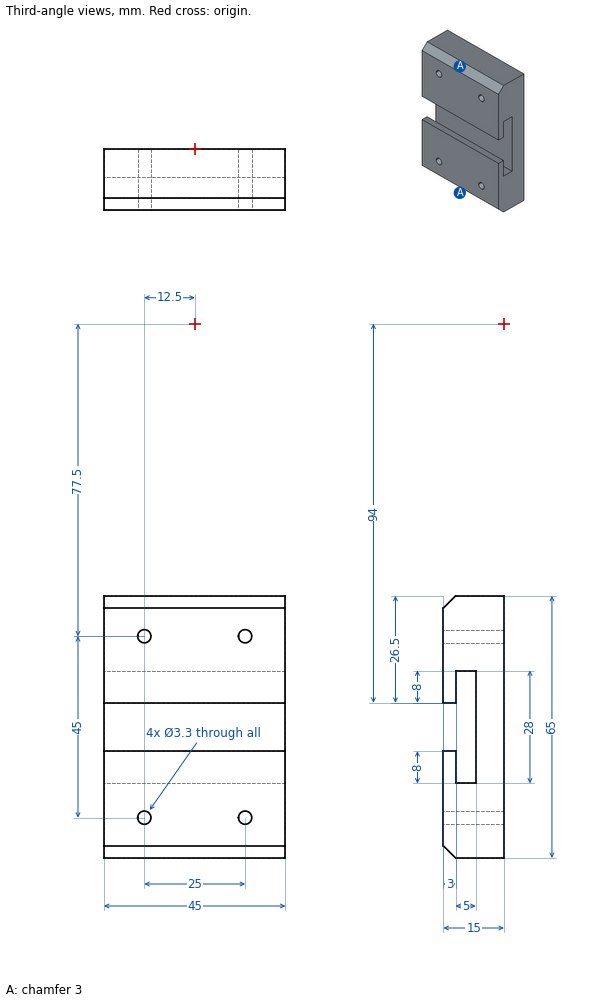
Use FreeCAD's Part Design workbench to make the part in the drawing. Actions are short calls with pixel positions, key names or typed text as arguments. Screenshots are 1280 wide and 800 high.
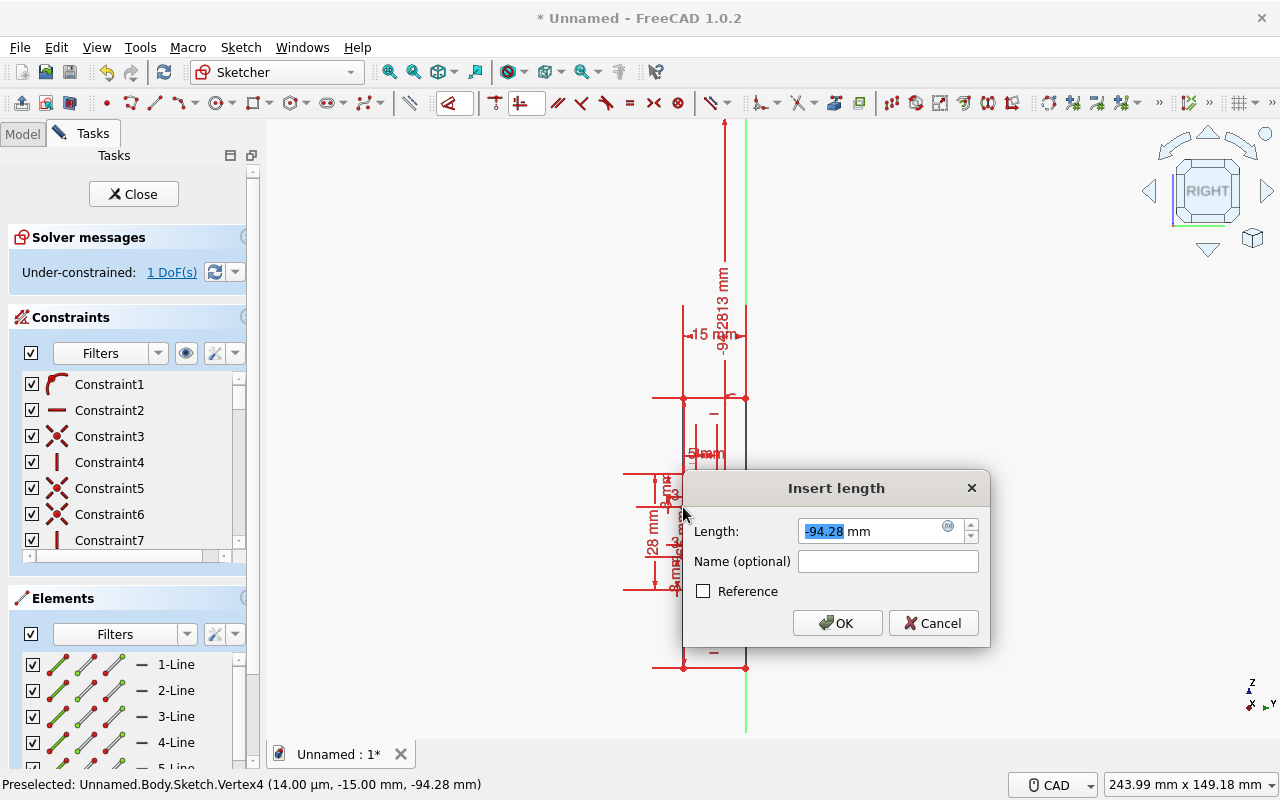
text(-94)
key(Return)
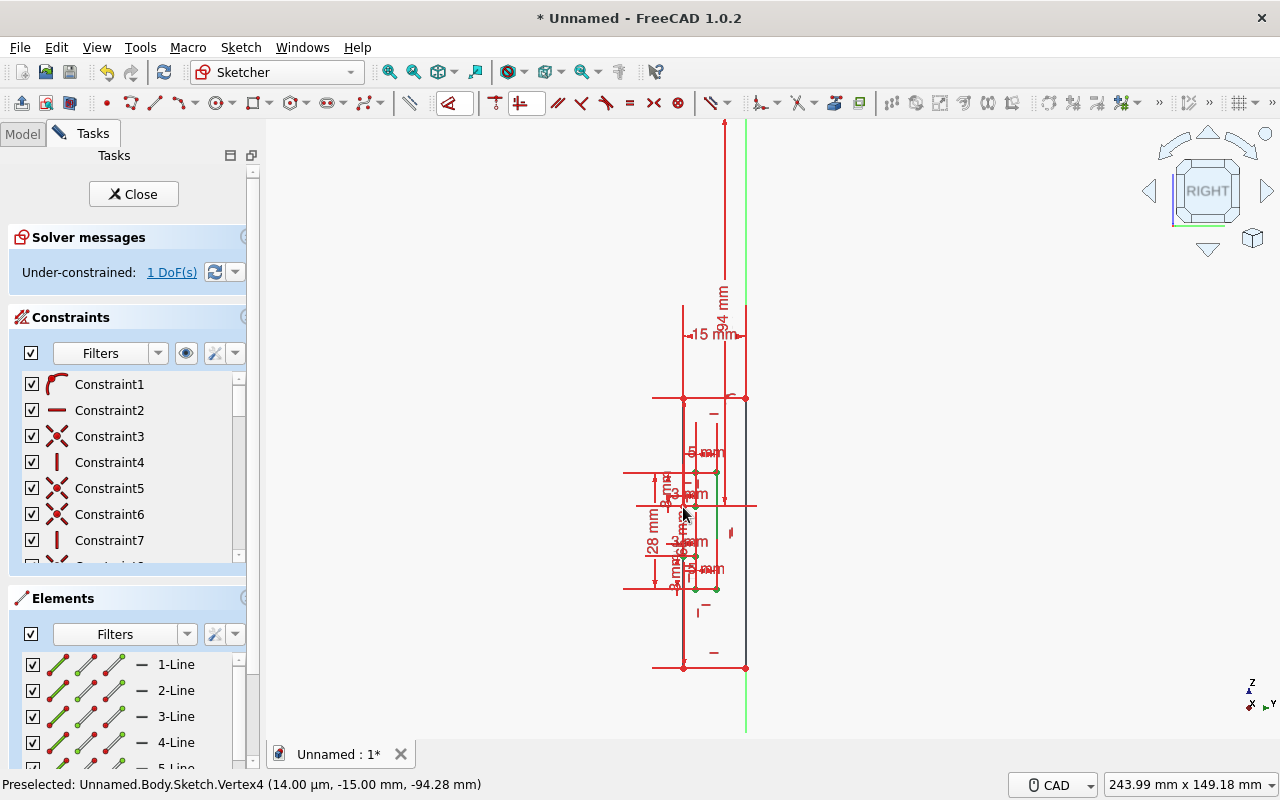
click(683, 431)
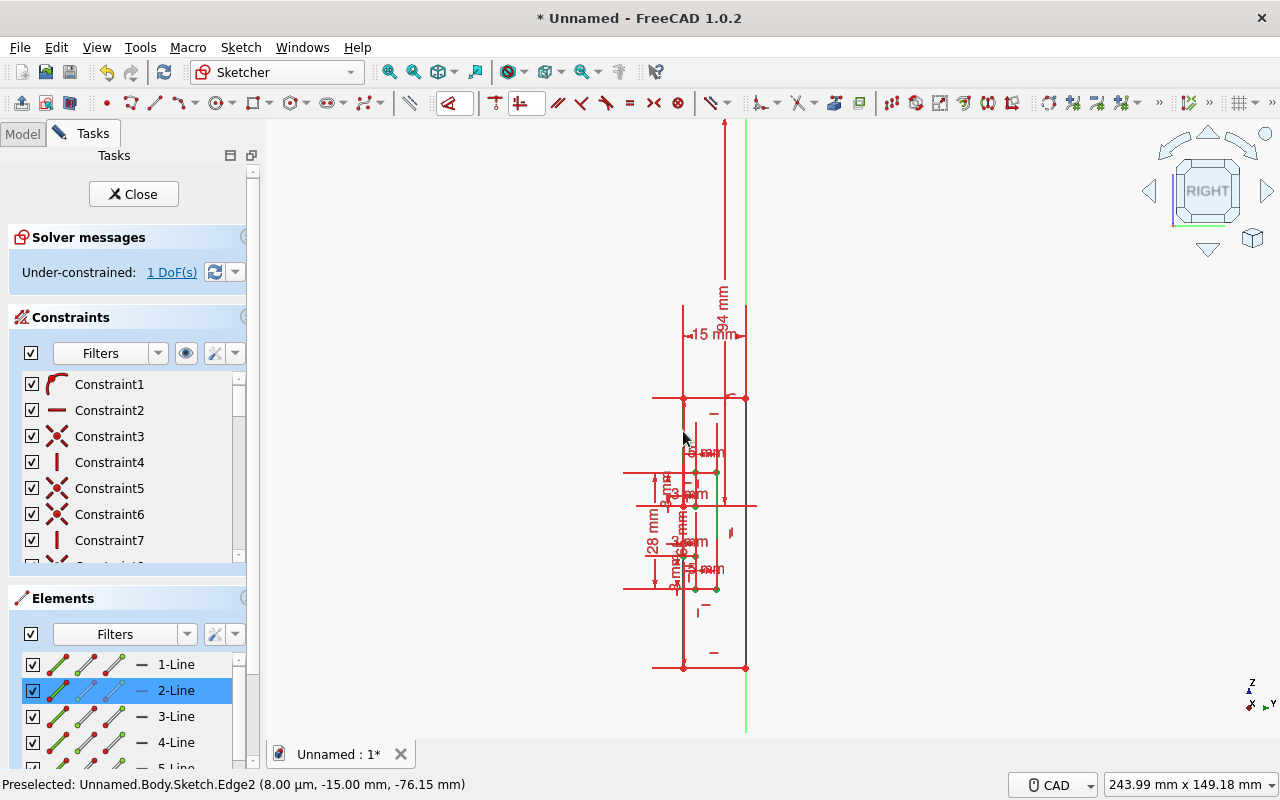
key(i)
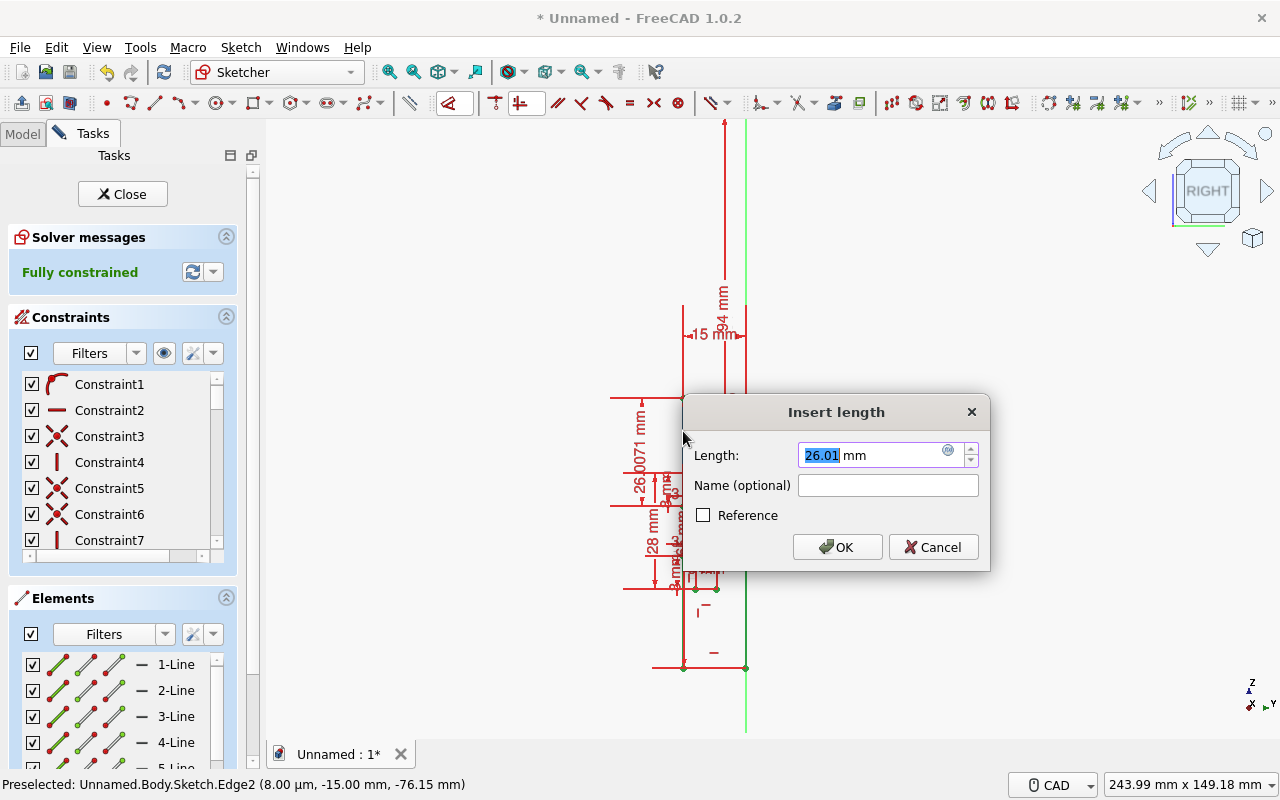
text(26.5)
key(Return)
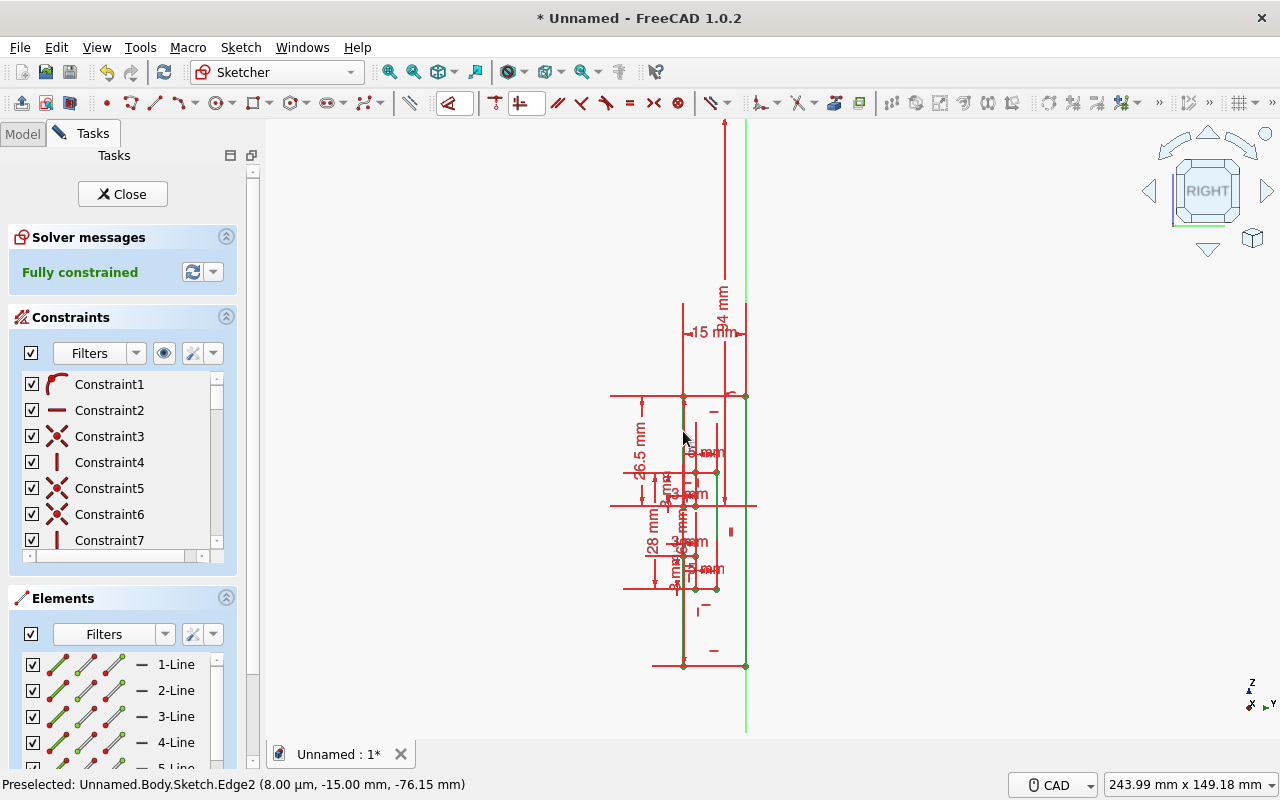
click(123, 194)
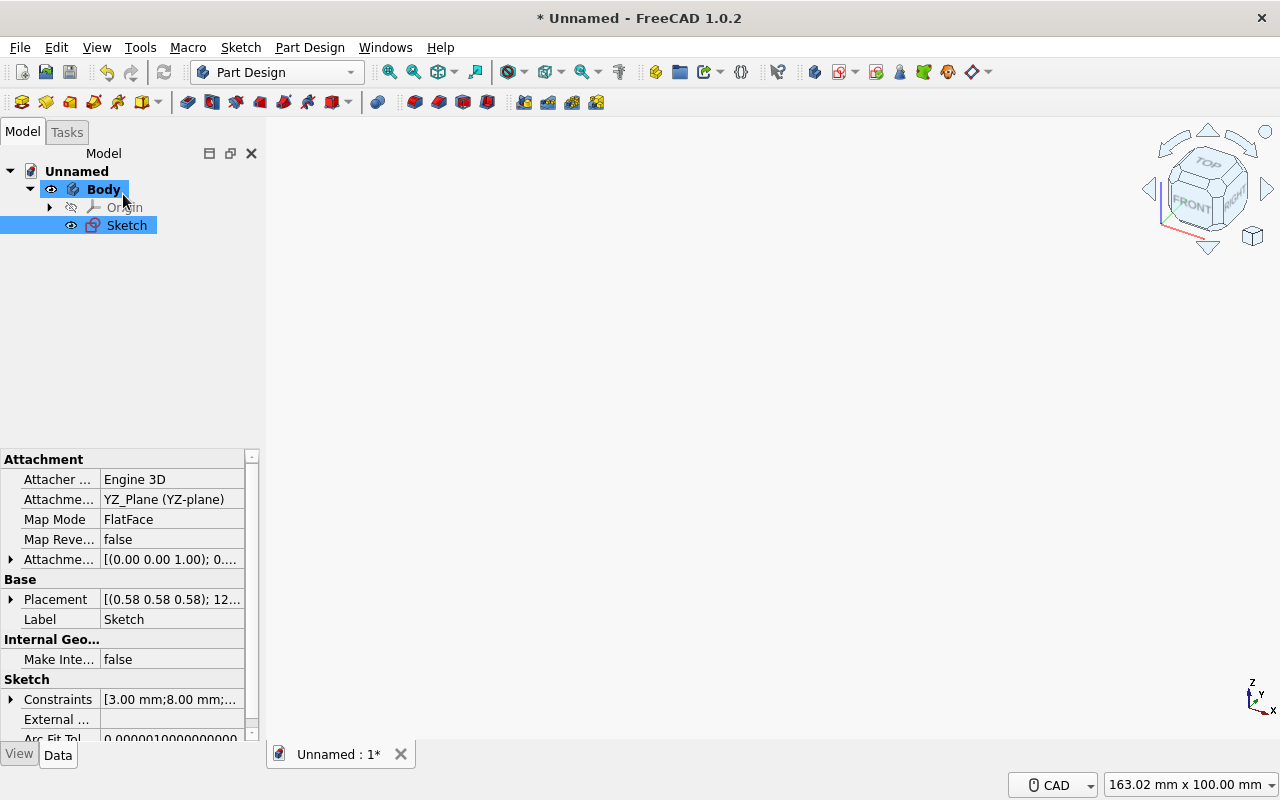
click(22, 102)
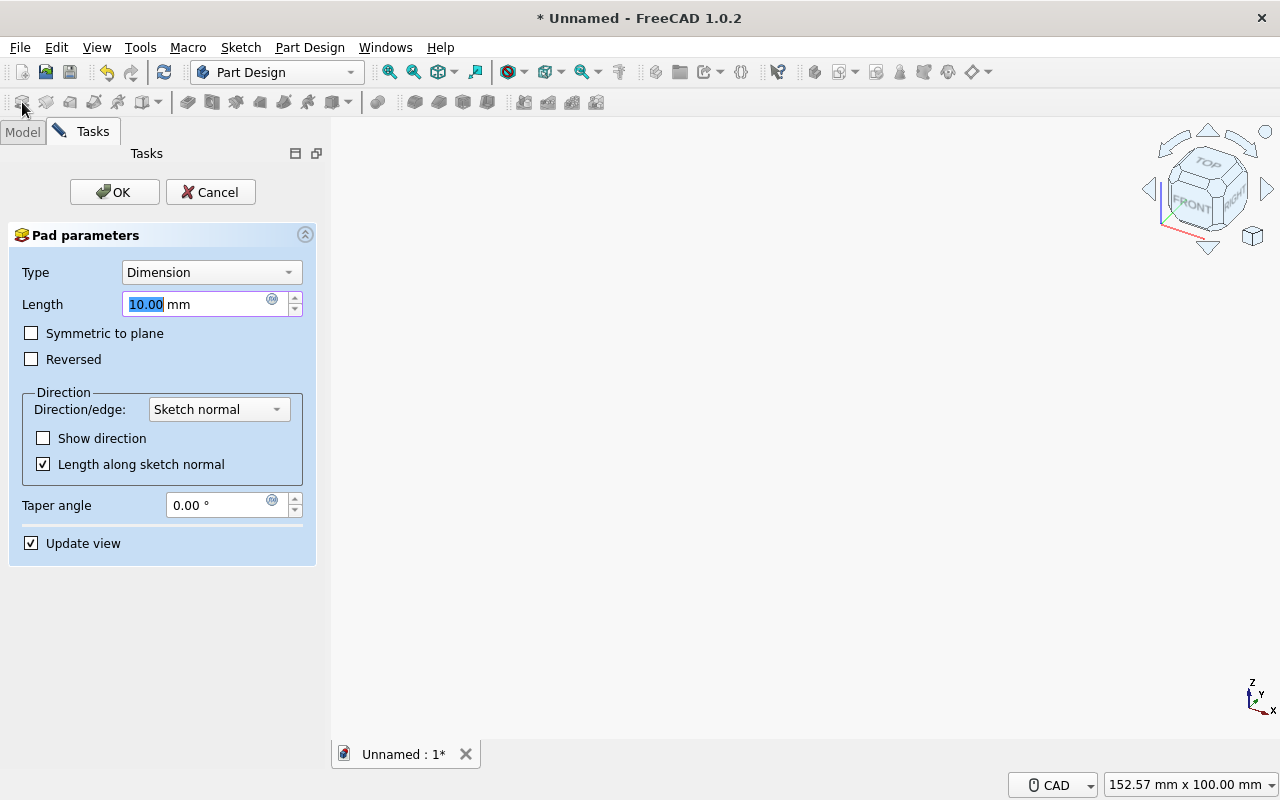
text(45)
key(Tab)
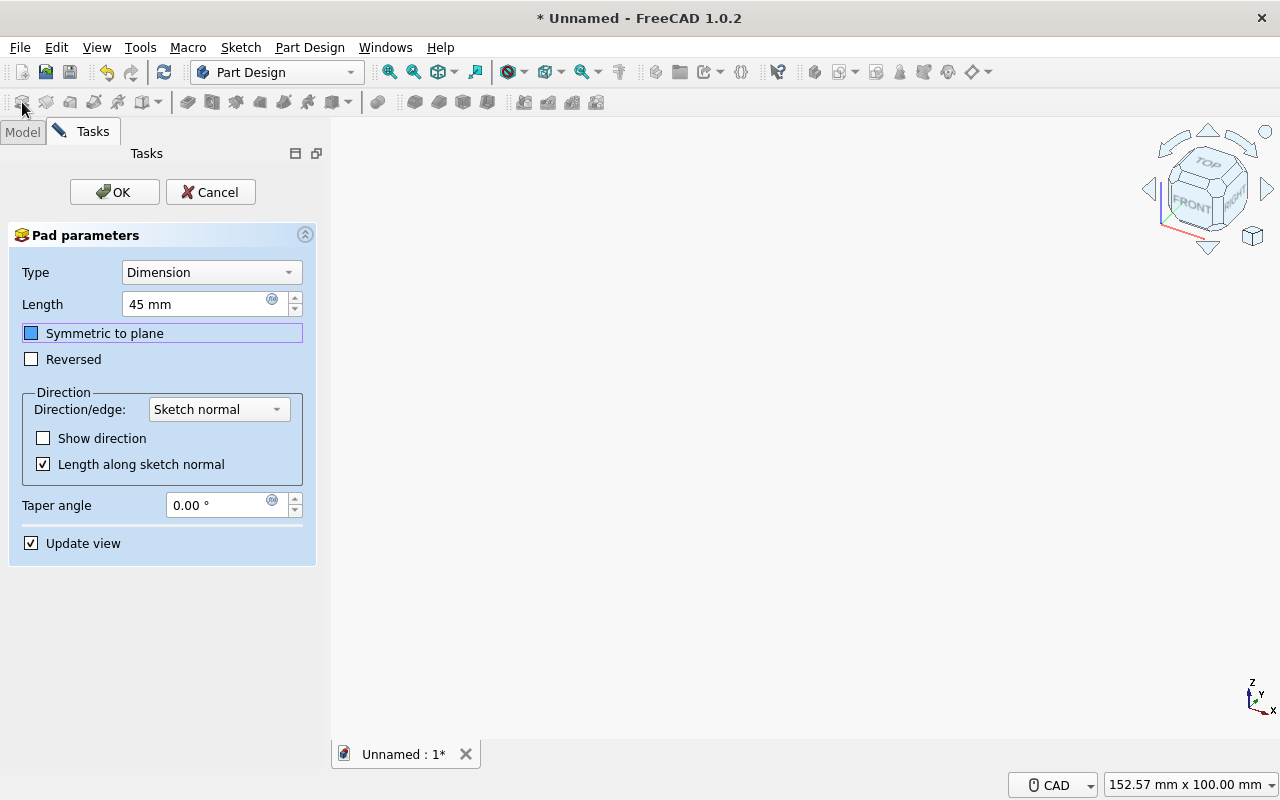
click(30, 333)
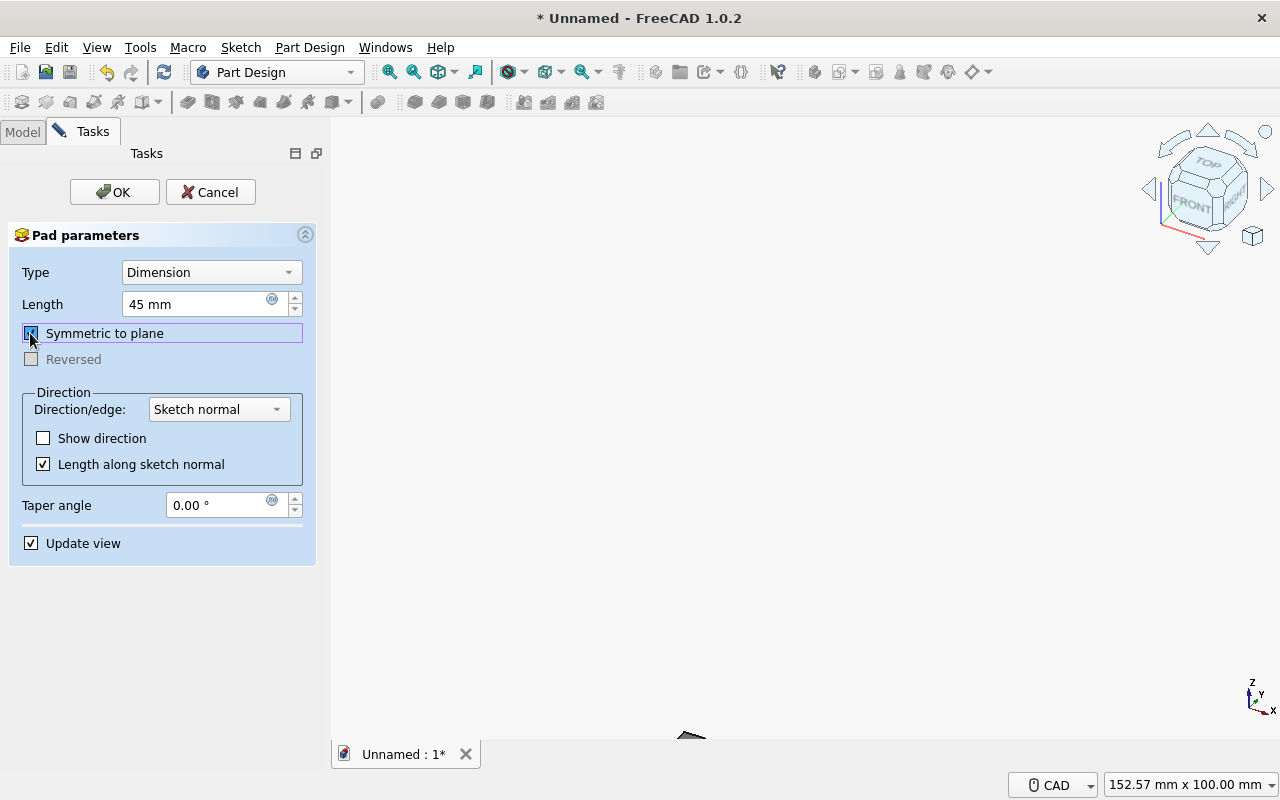
click(115, 192)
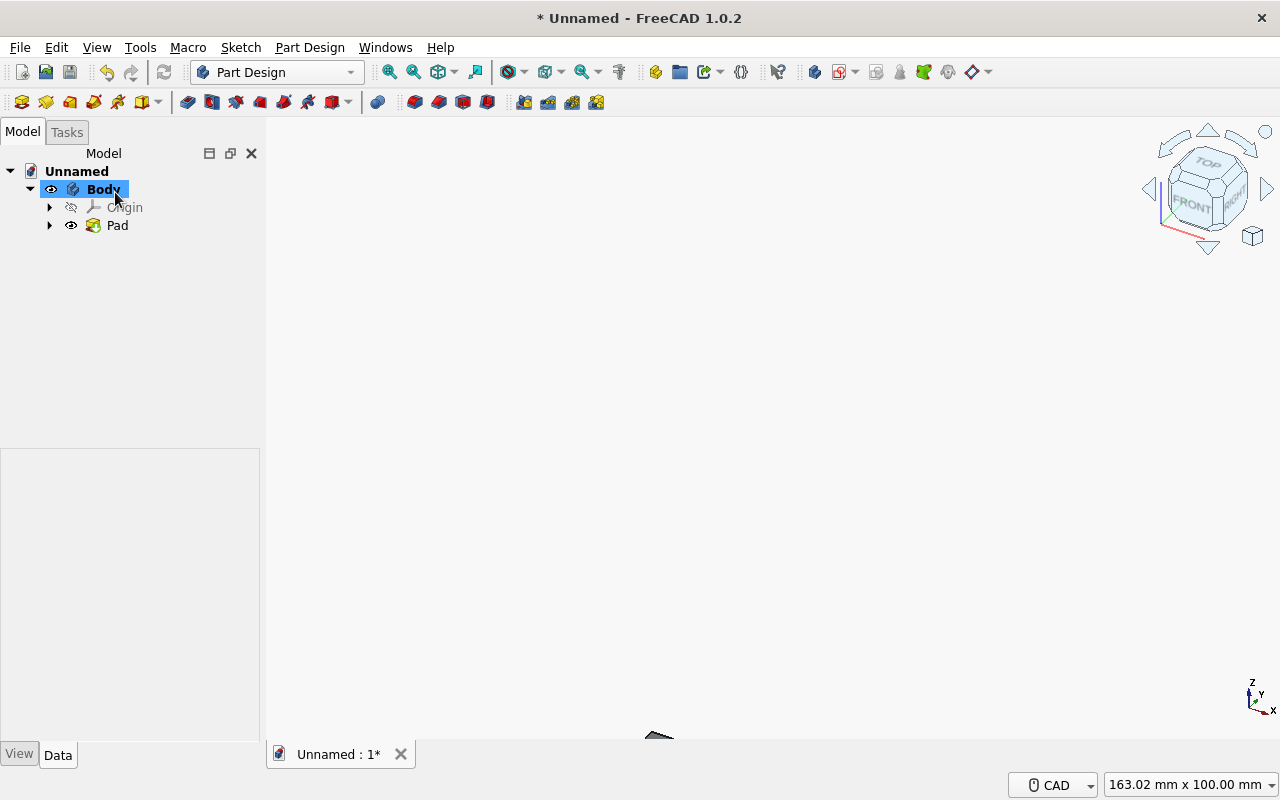
click(390, 72)